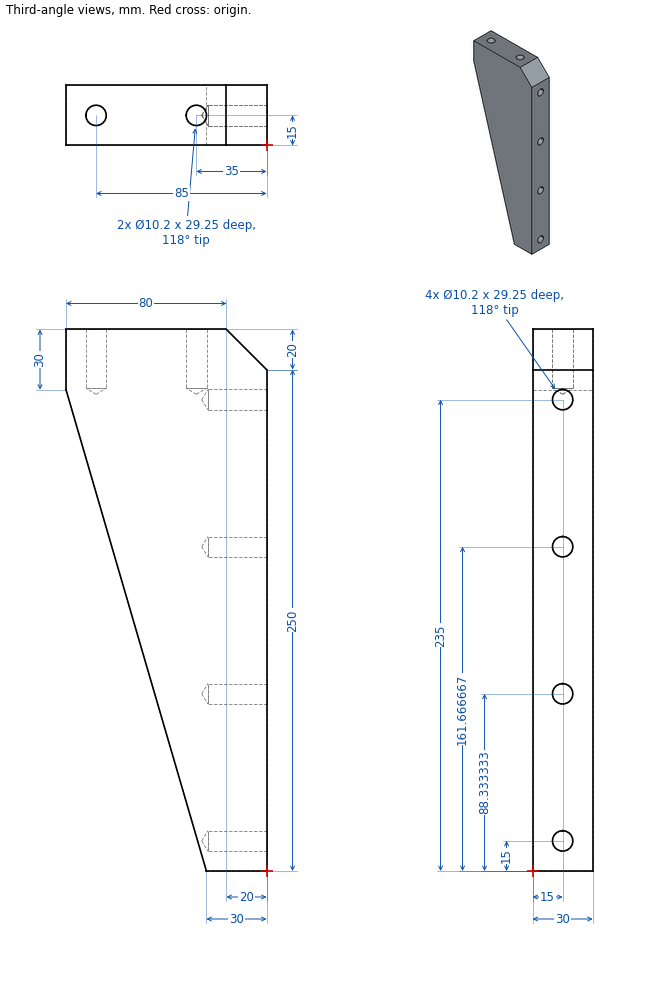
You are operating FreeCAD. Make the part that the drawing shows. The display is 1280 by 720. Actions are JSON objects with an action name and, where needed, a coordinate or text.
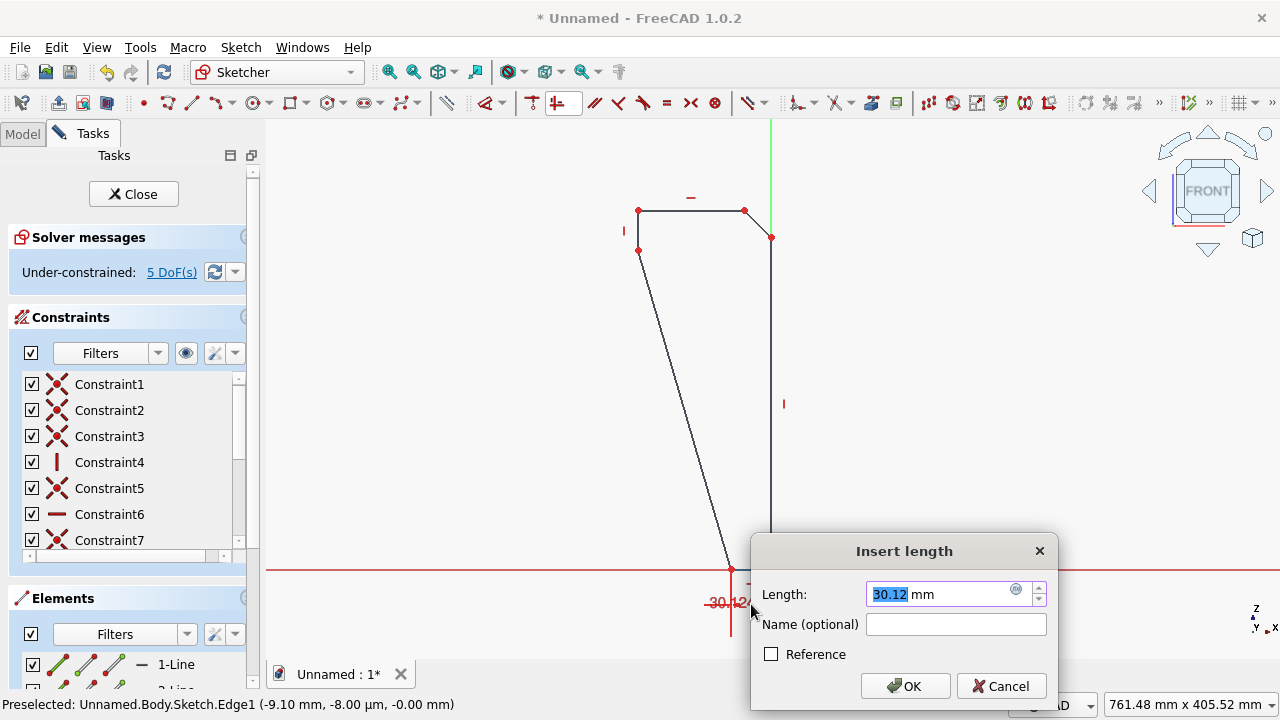
{"action": "type", "text": "30"}
{"action": "key", "text": "Return"}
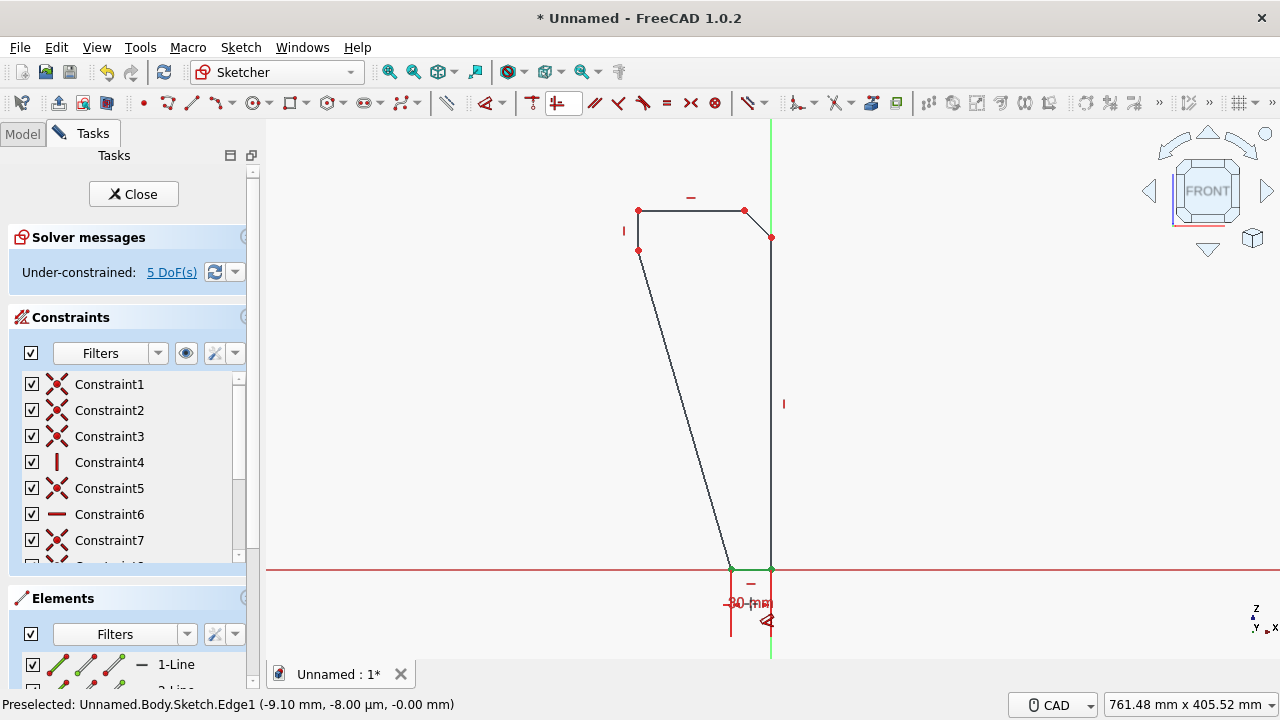
{"action": "left_click", "coordinate": [638, 239]}
{"action": "left_click", "coordinate": [604, 231]}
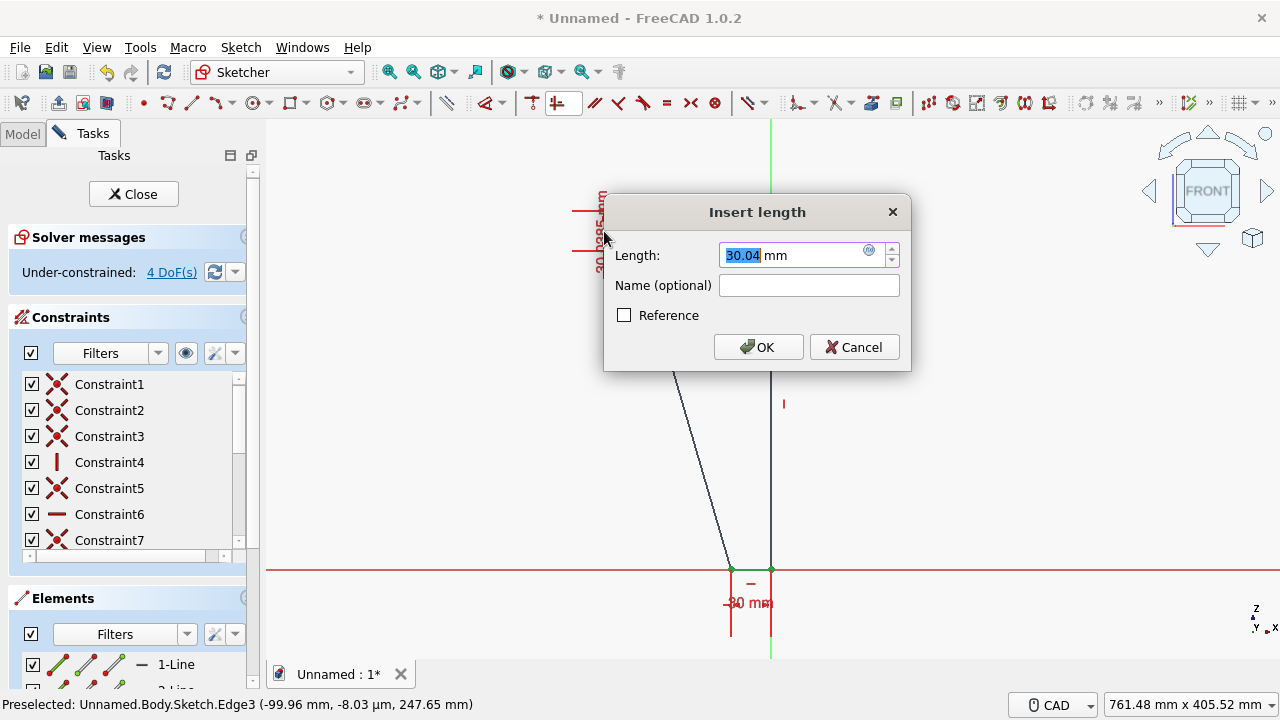
{"action": "type", "text": "30"}
{"action": "key", "text": "Return"}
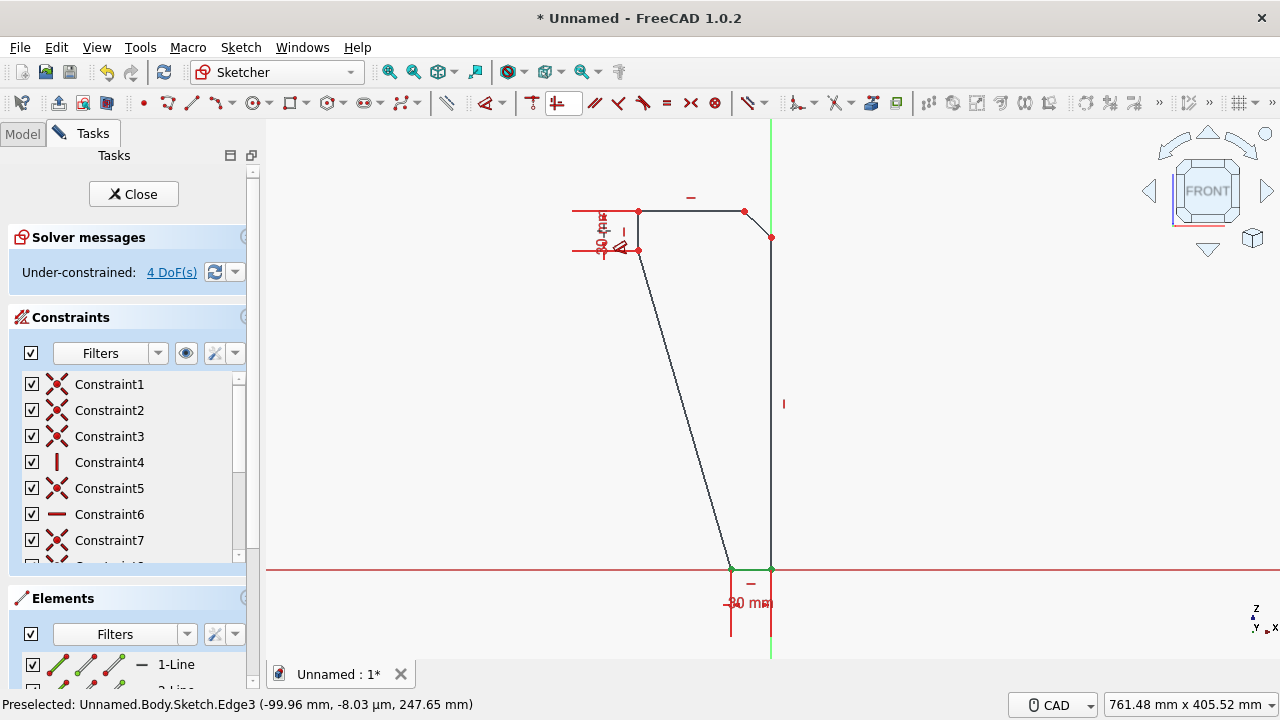
{"action": "left_click", "coordinate": [670, 211]}
{"action": "left_click", "coordinate": [691, 177]}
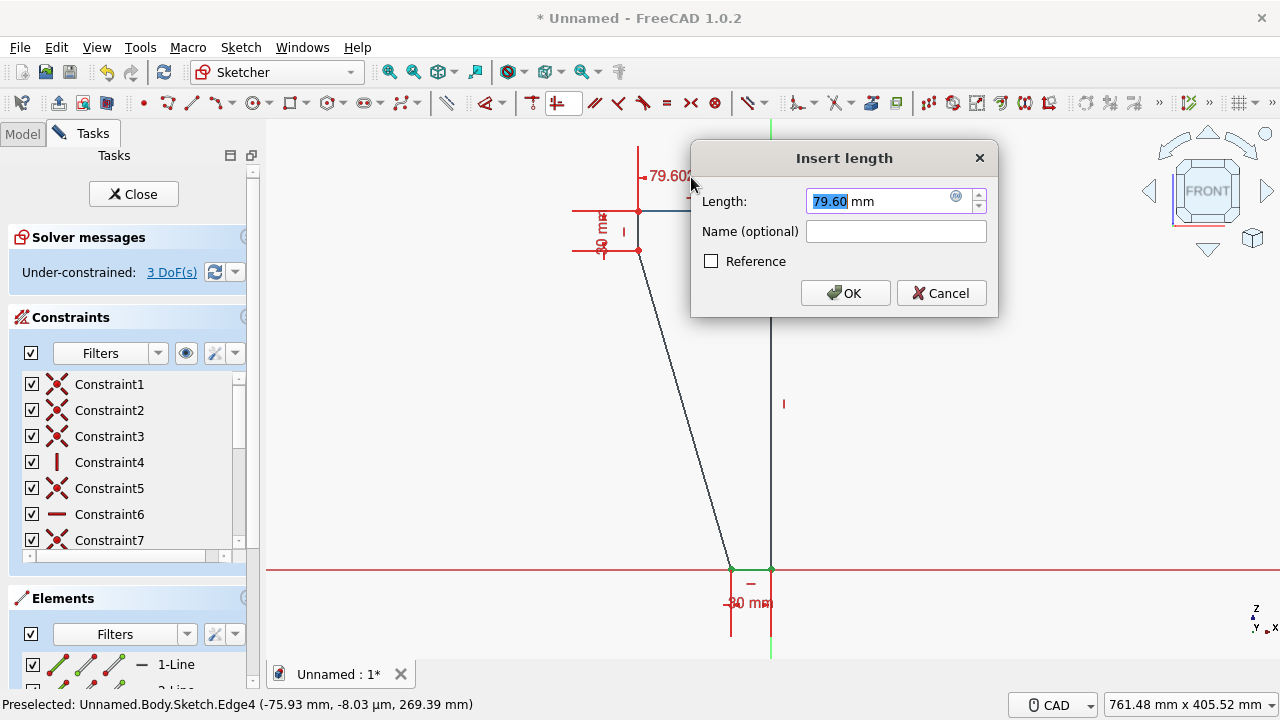
{"action": "type", "text": "80"}
{"action": "key", "text": "Return"}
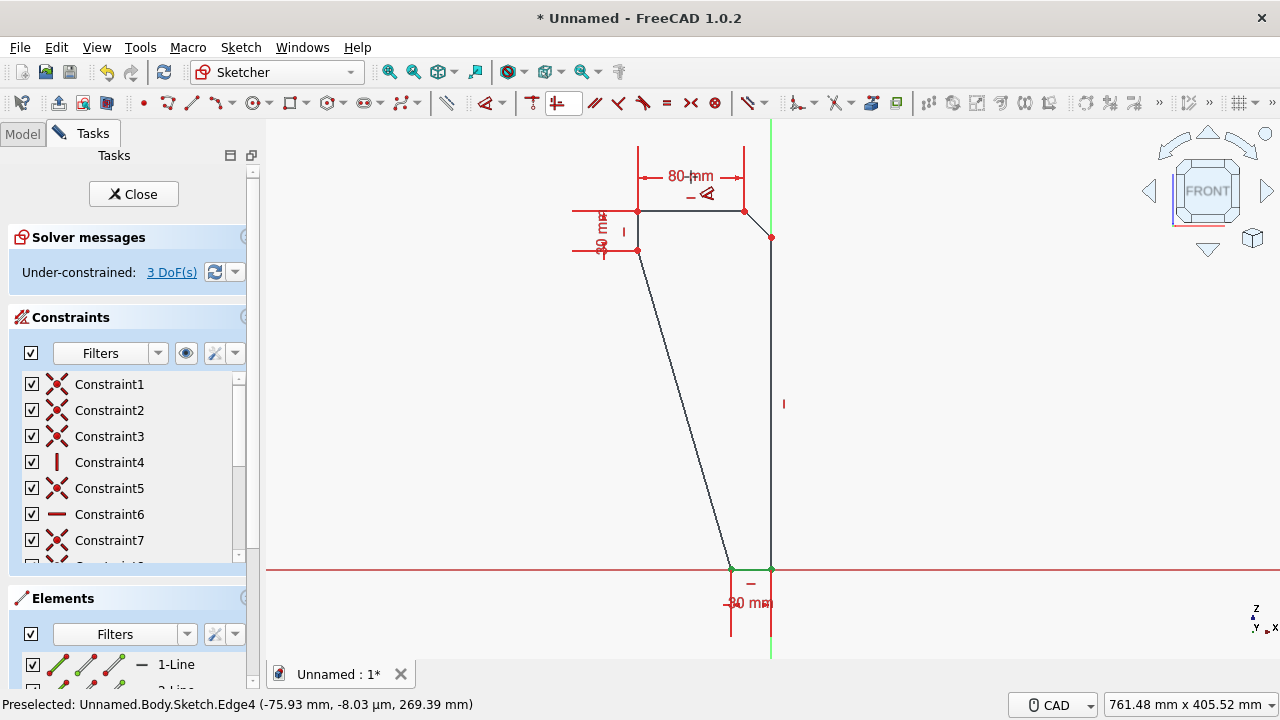
{"action": "left_click", "coordinate": [771, 338]}
{"action": "left_click", "coordinate": [805, 404]}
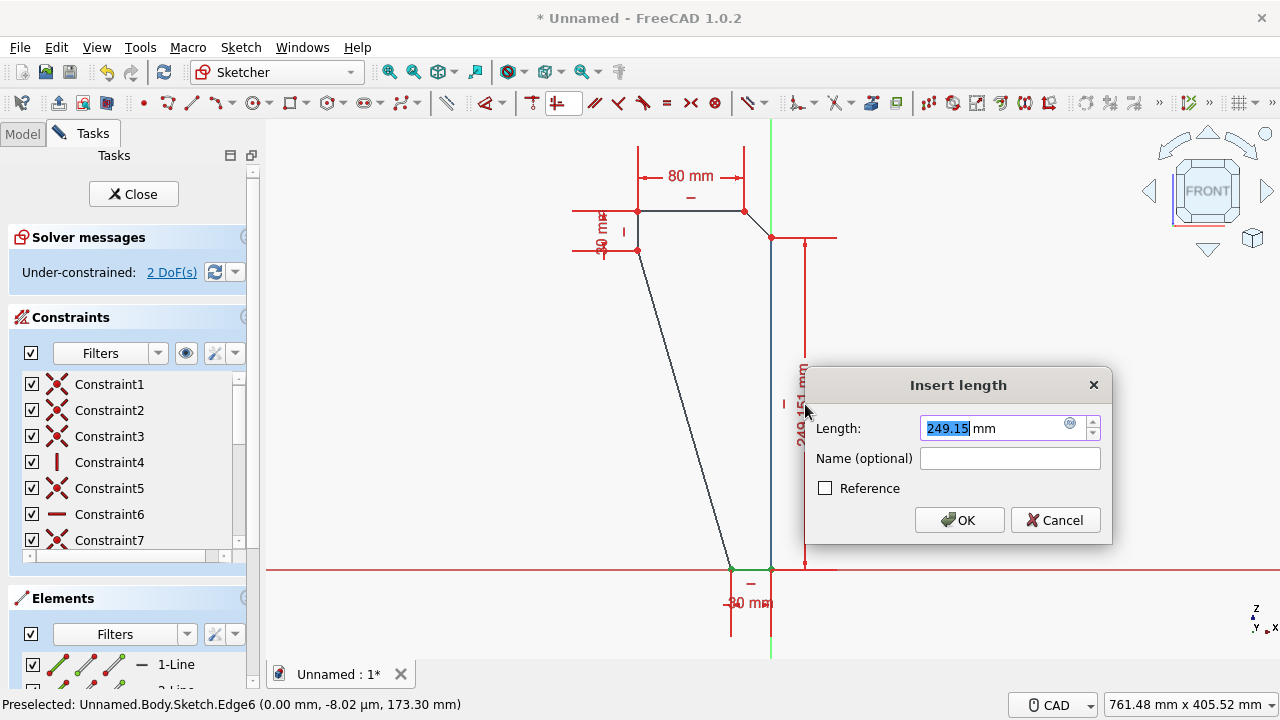
{"action": "type", "text": "250"}
{"action": "key", "text": "Return"}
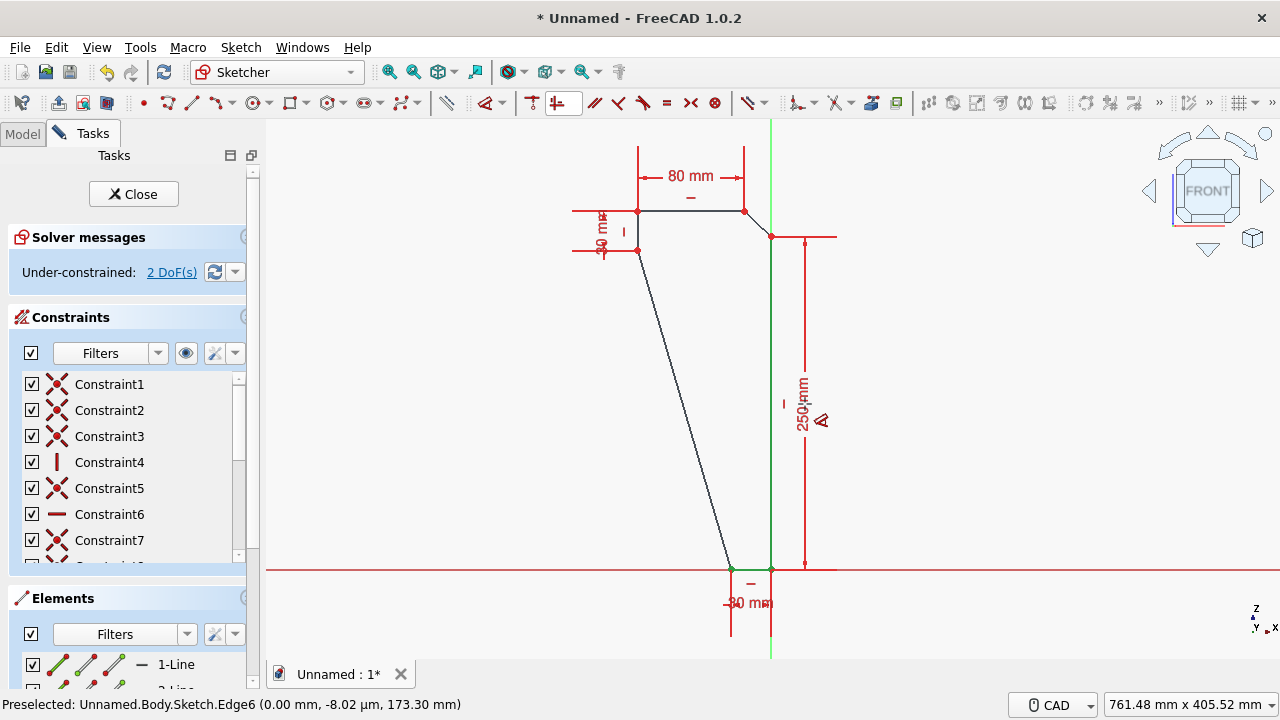
{"action": "scroll", "coordinate": [744, 211], "scroll_direction": "up", "scroll_amount": 2}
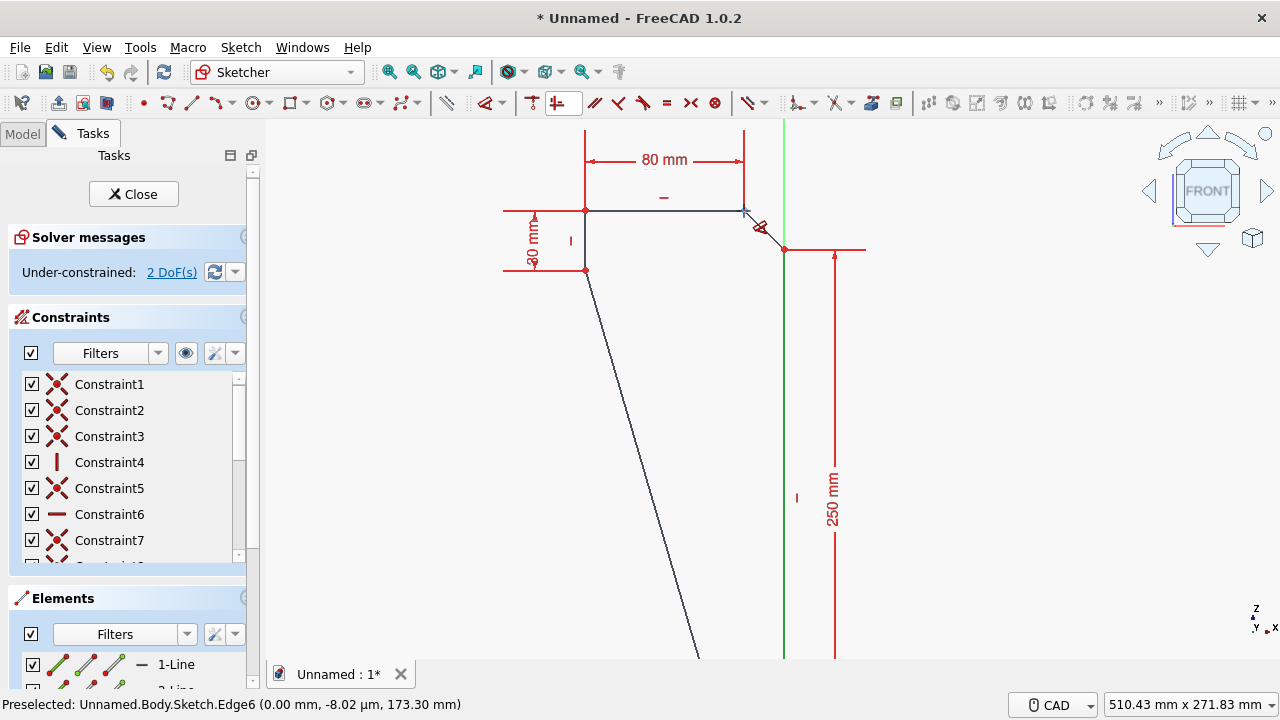
{"action": "left_click", "coordinate": [744, 211]}
{"action": "left_click", "coordinate": [764, 177]}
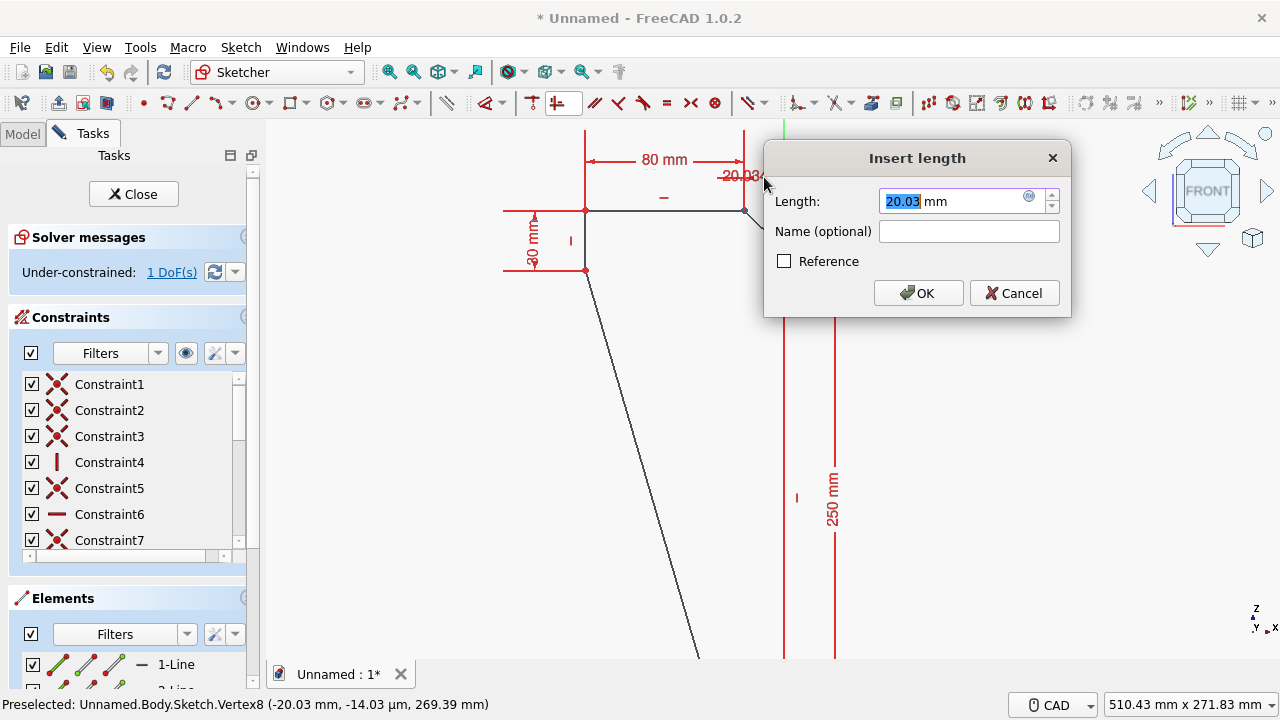
{"action": "type", "text": "20"}
{"action": "key", "text": "Return"}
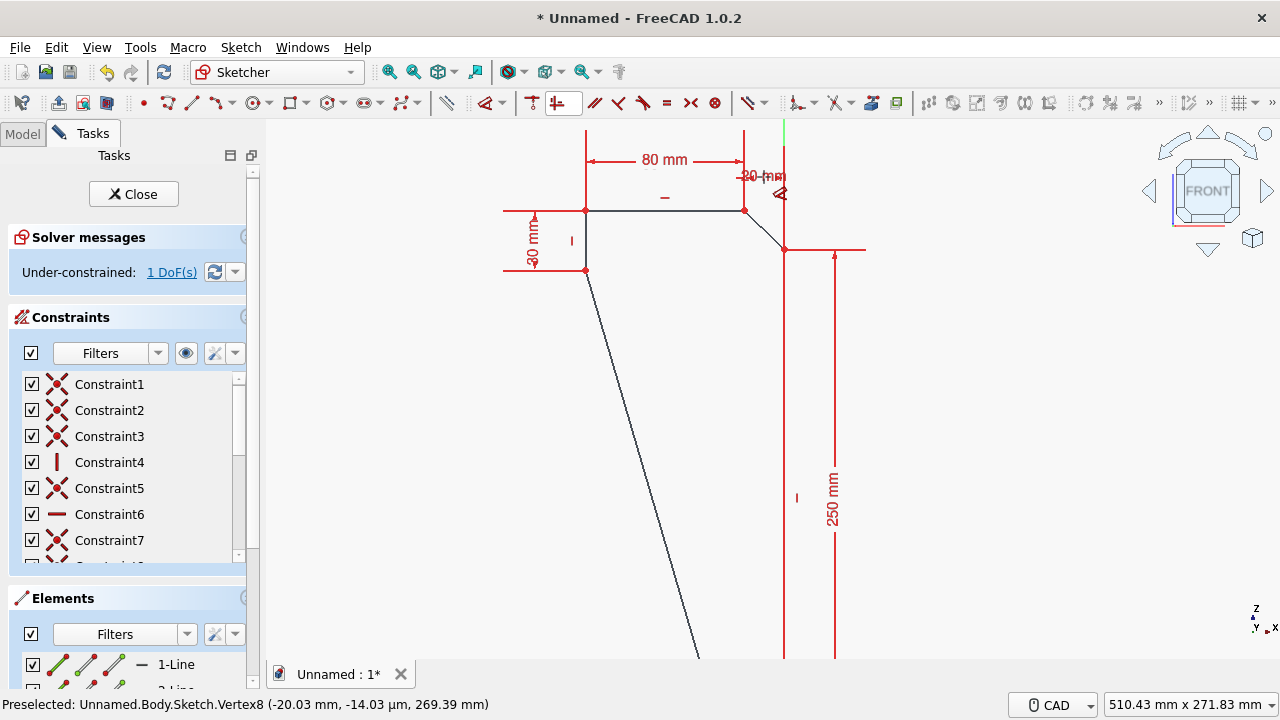
{"action": "left_click", "coordinate": [756, 223]}
{"action": "left_click", "coordinate": [818, 230]}